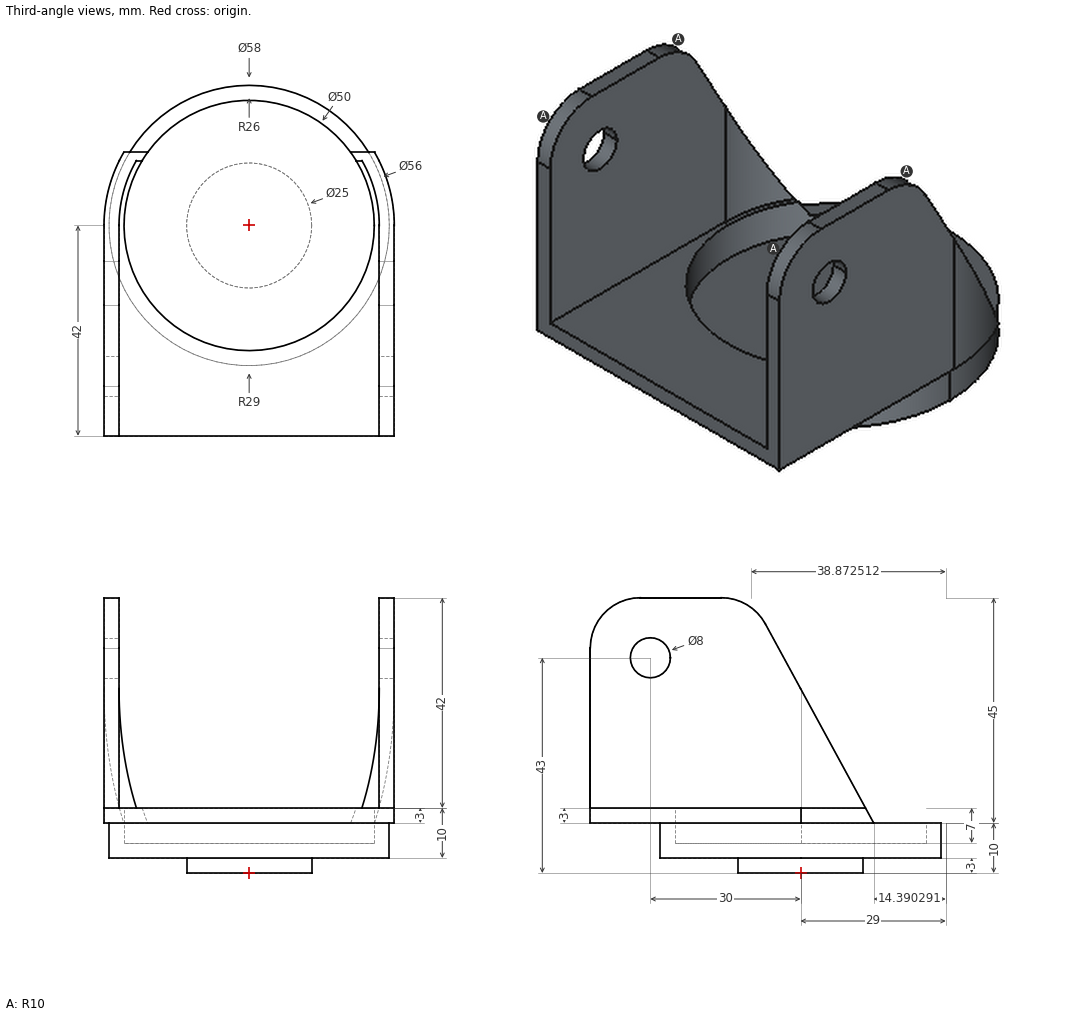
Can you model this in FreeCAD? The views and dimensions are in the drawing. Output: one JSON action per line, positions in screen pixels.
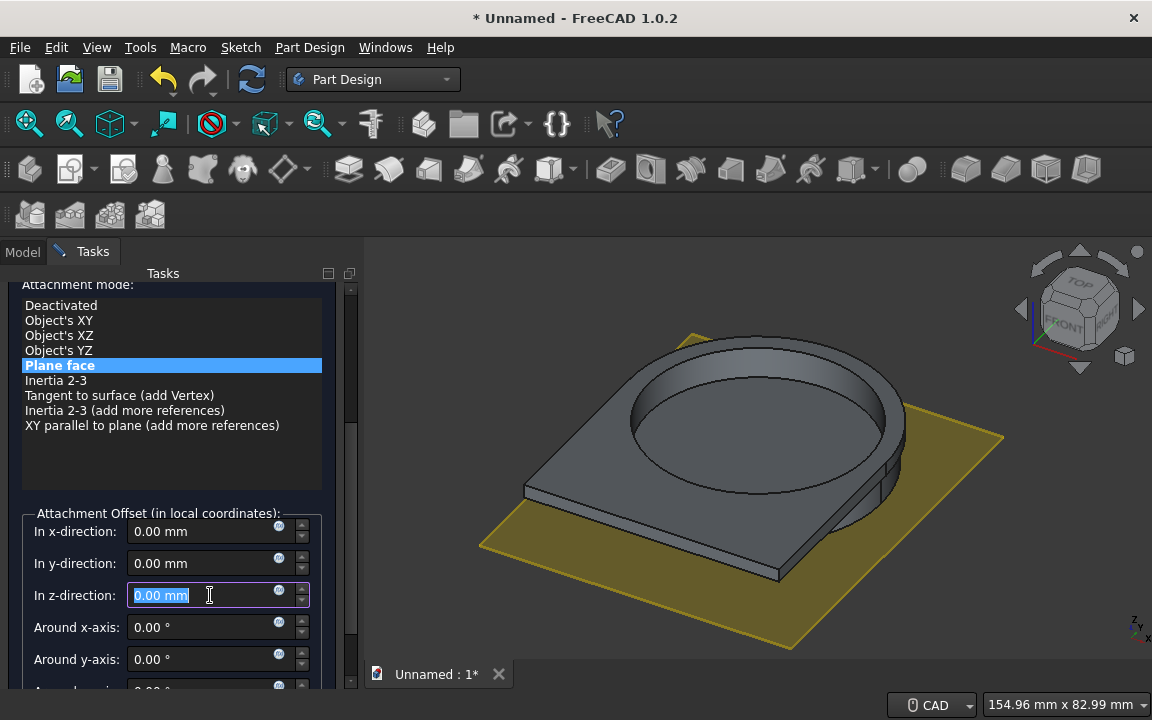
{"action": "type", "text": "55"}
{"action": "key", "text": "Tab"}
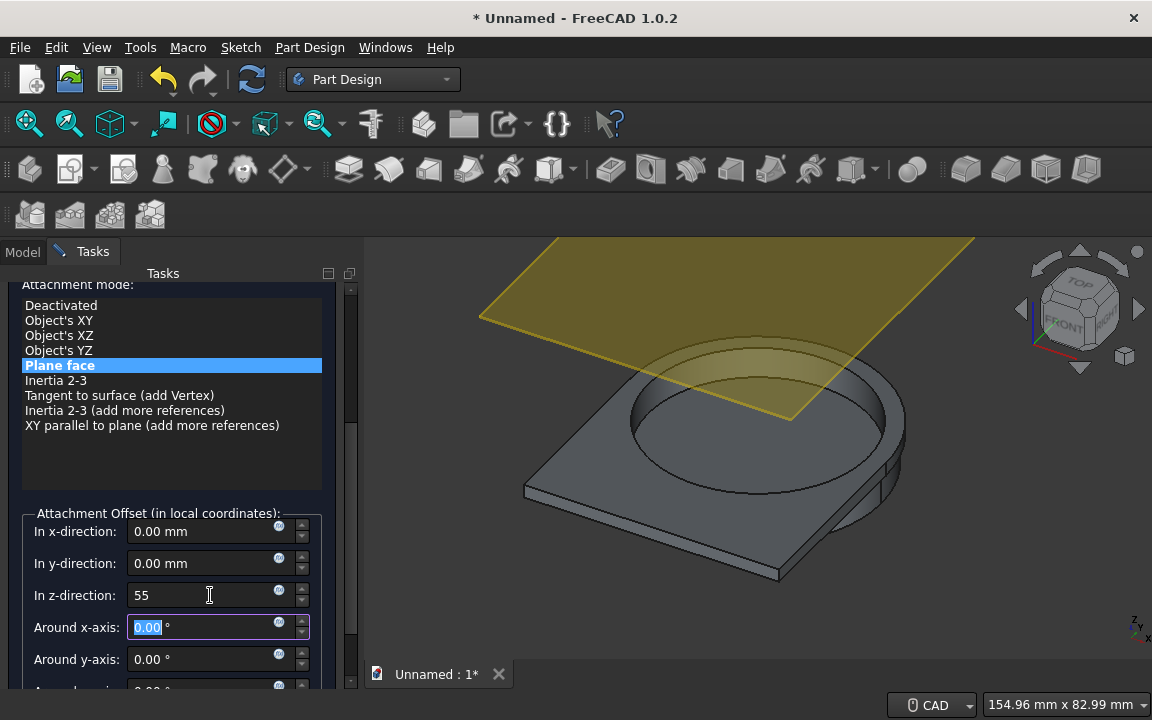
{"action": "scroll", "coordinate": [351, 486], "scroll_direction": "up", "scroll_amount": 5}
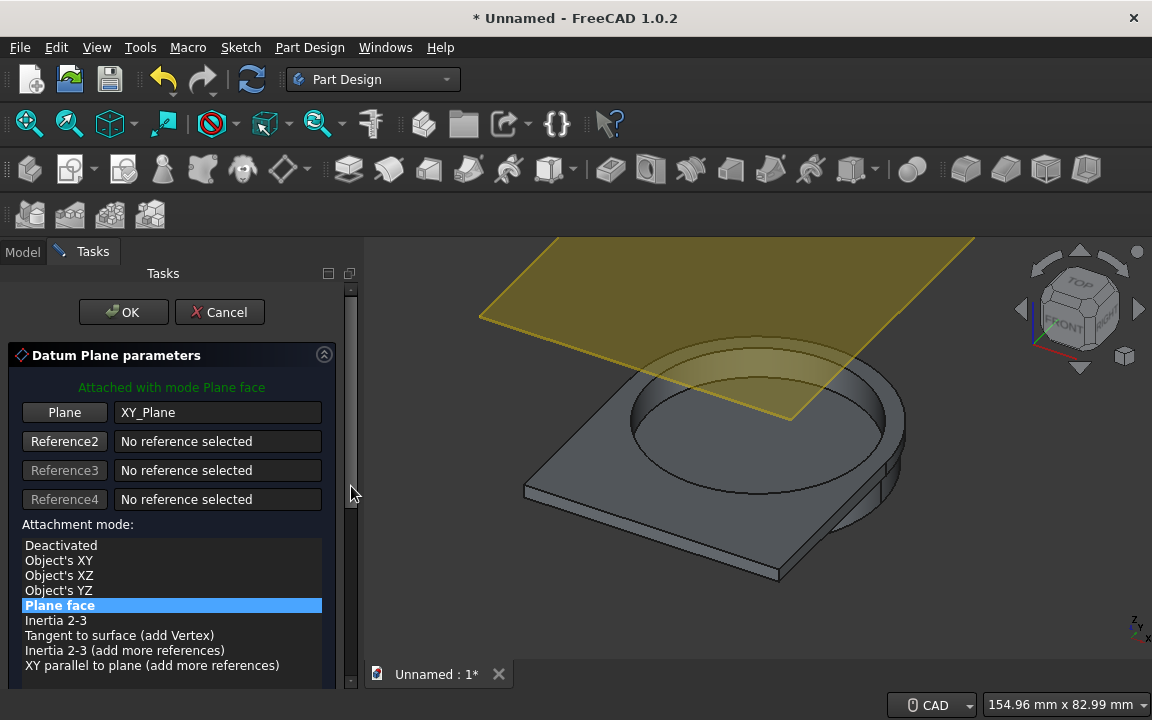
{"action": "left_click", "coordinate": [124, 312]}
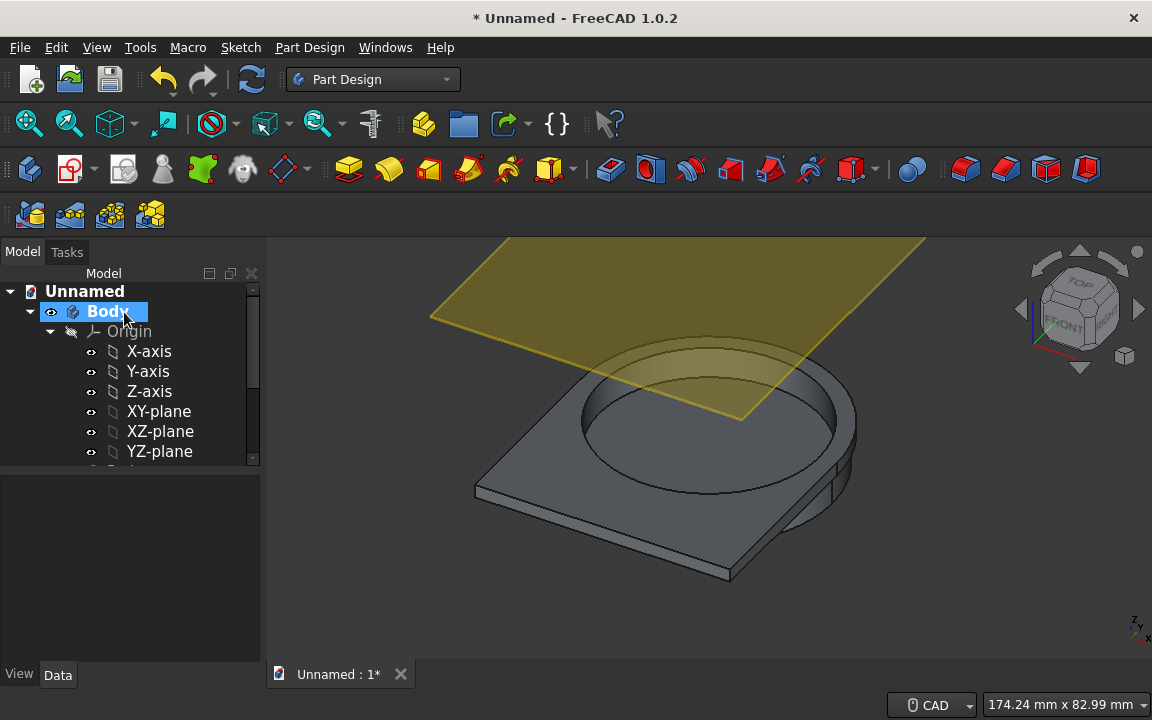
{"action": "scroll", "coordinate": [100, 367], "scroll_direction": "down", "scroll_amount": 3}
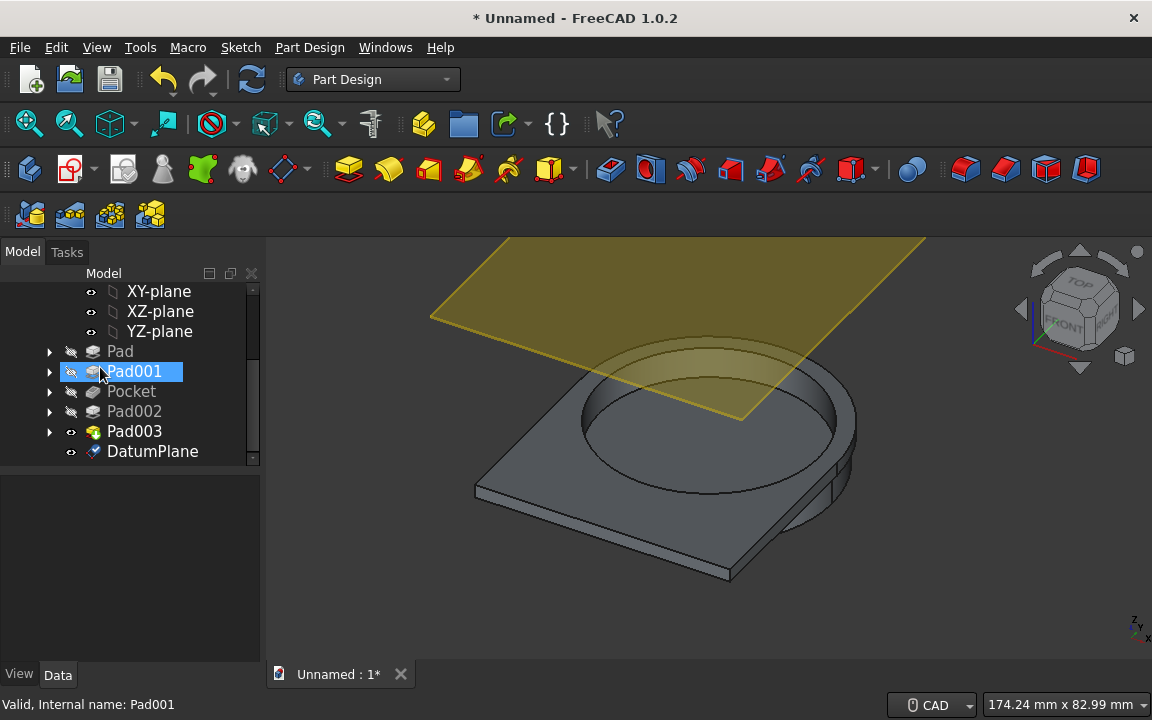
{"action": "left_click", "coordinate": [116, 452]}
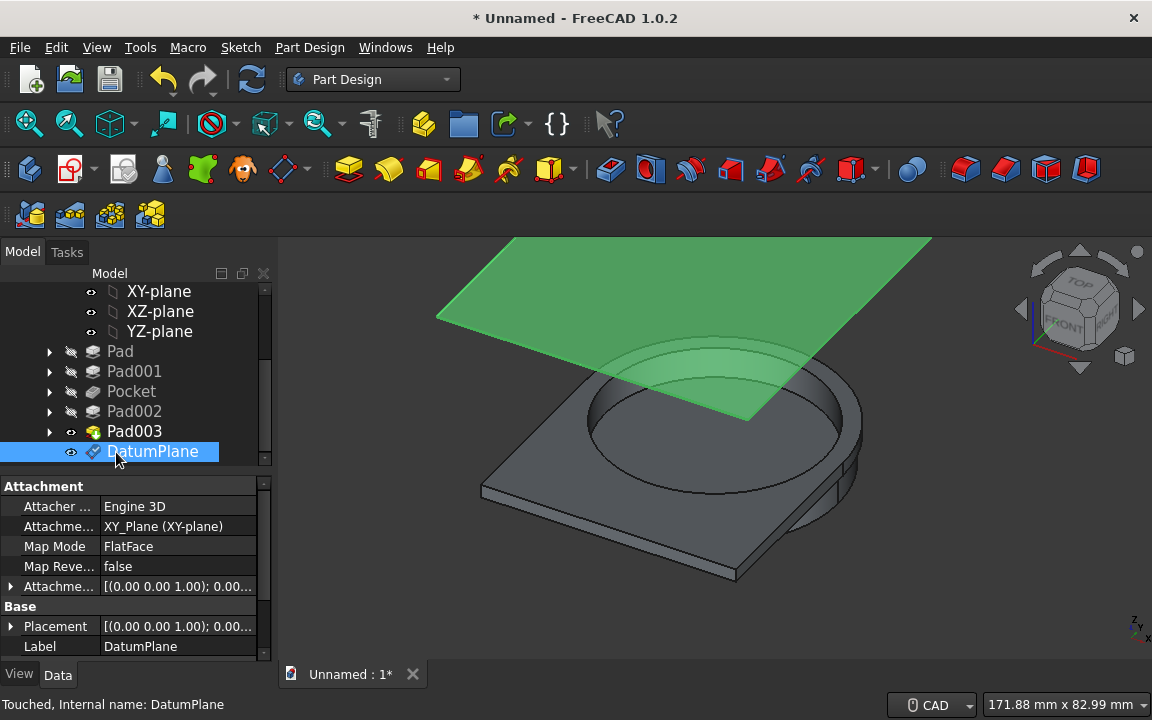
{"action": "left_click", "coordinate": [70, 170]}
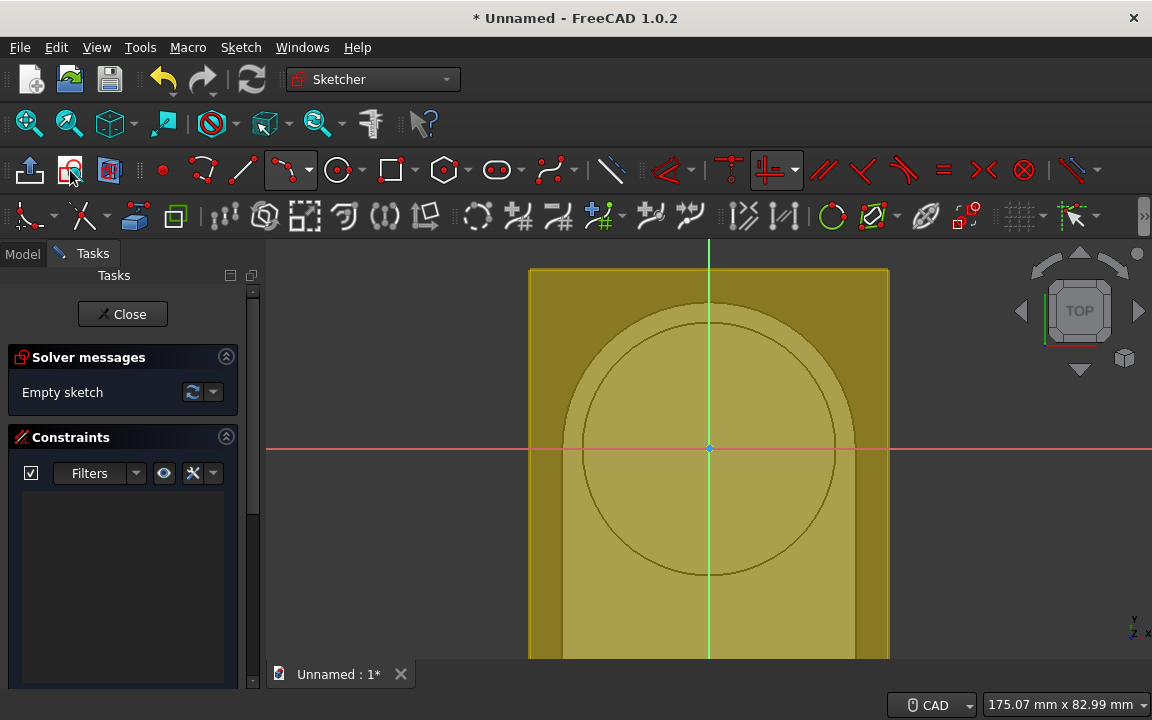
{"action": "scroll", "coordinate": [501, 382], "scroll_direction": "down", "scroll_amount": 2}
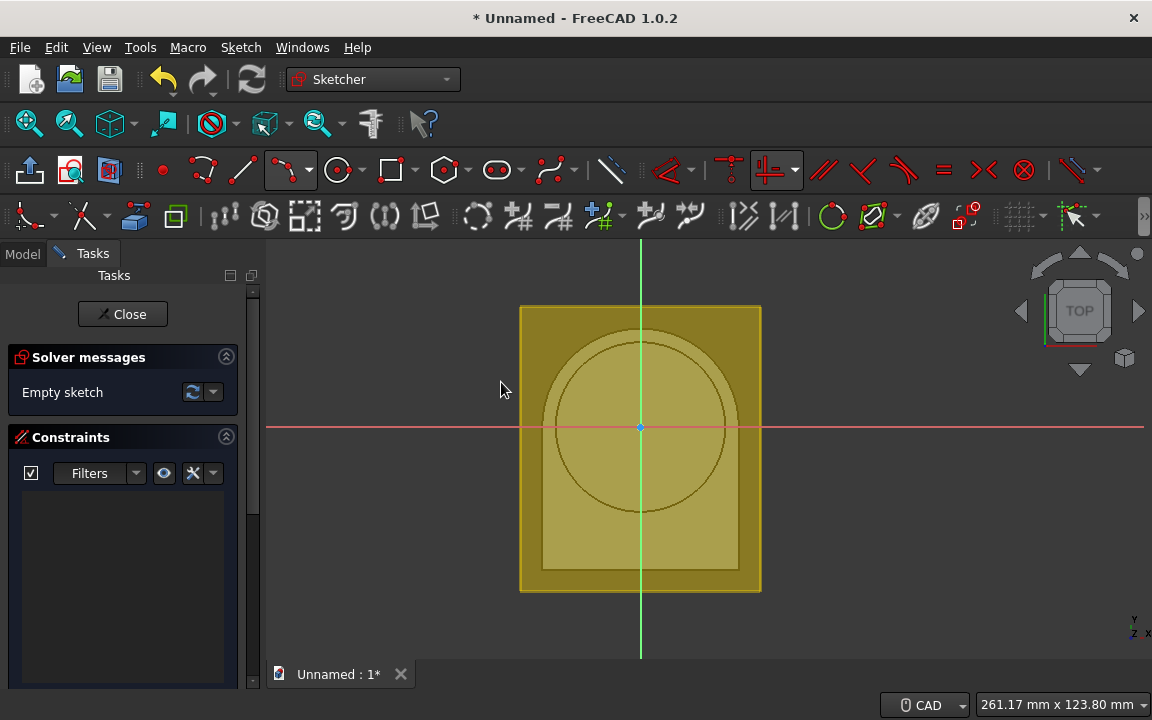
{"action": "left_click", "coordinate": [204, 170]}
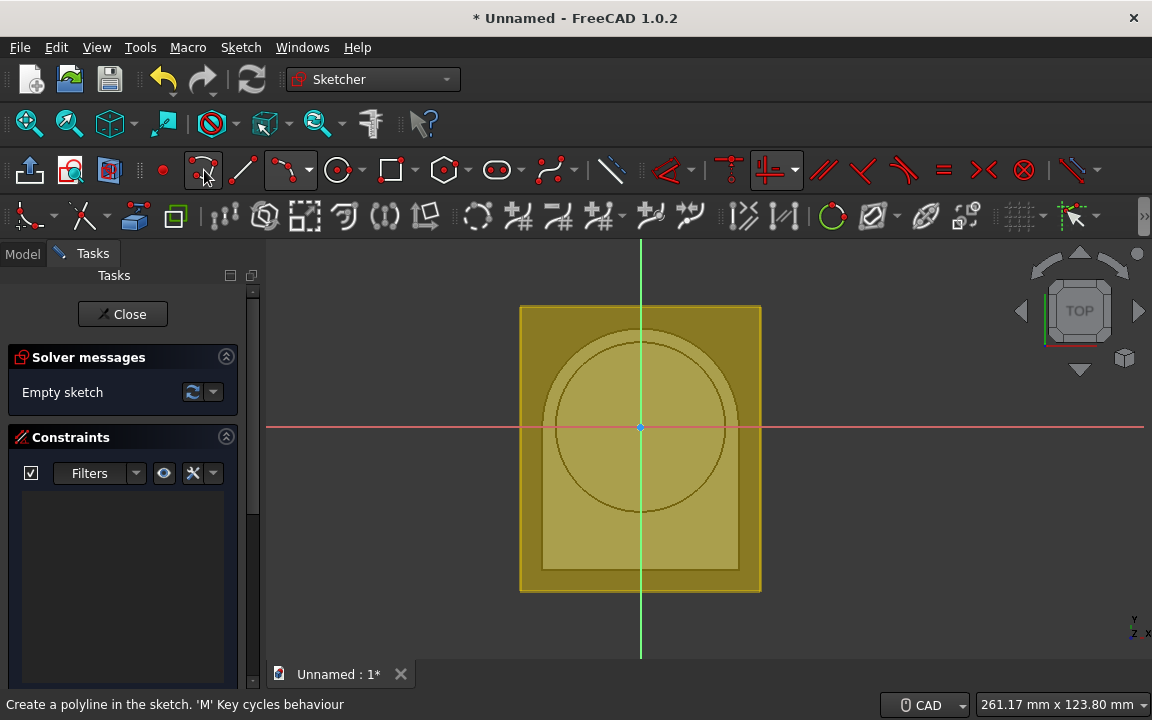
{"action": "left_click", "coordinate": [729, 427]}
{"action": "left_click", "coordinate": [729, 570]}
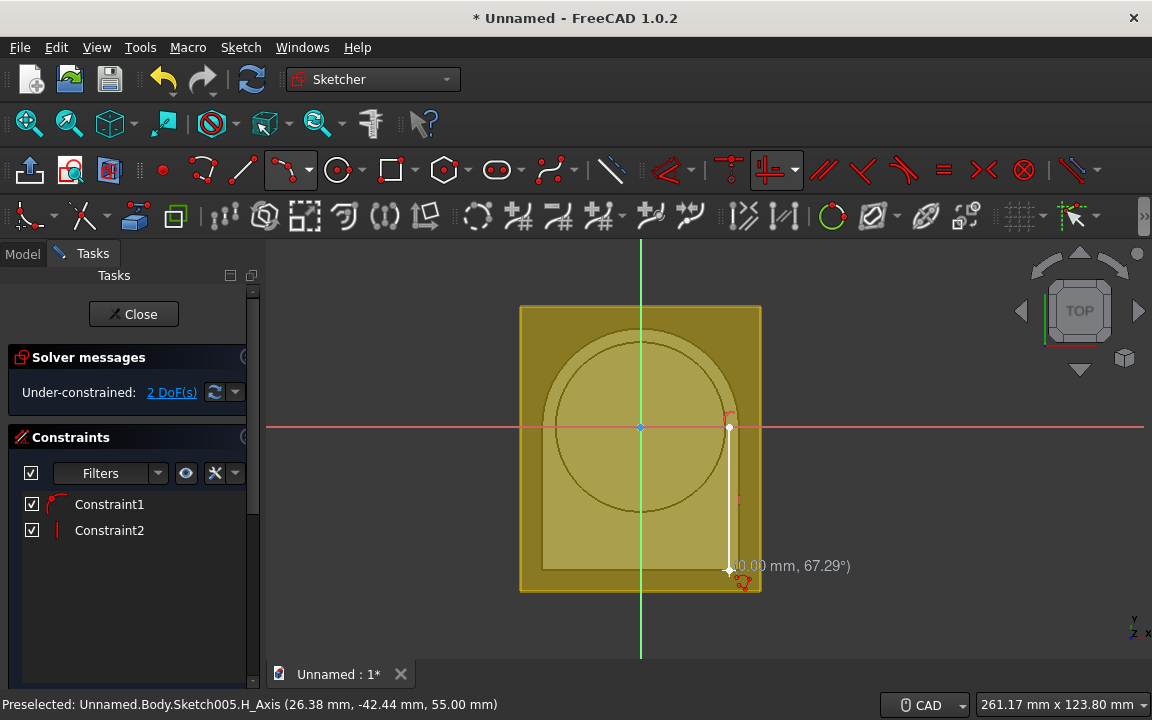
{"action": "scroll", "coordinate": [739, 570], "scroll_direction": "up", "scroll_amount": 3}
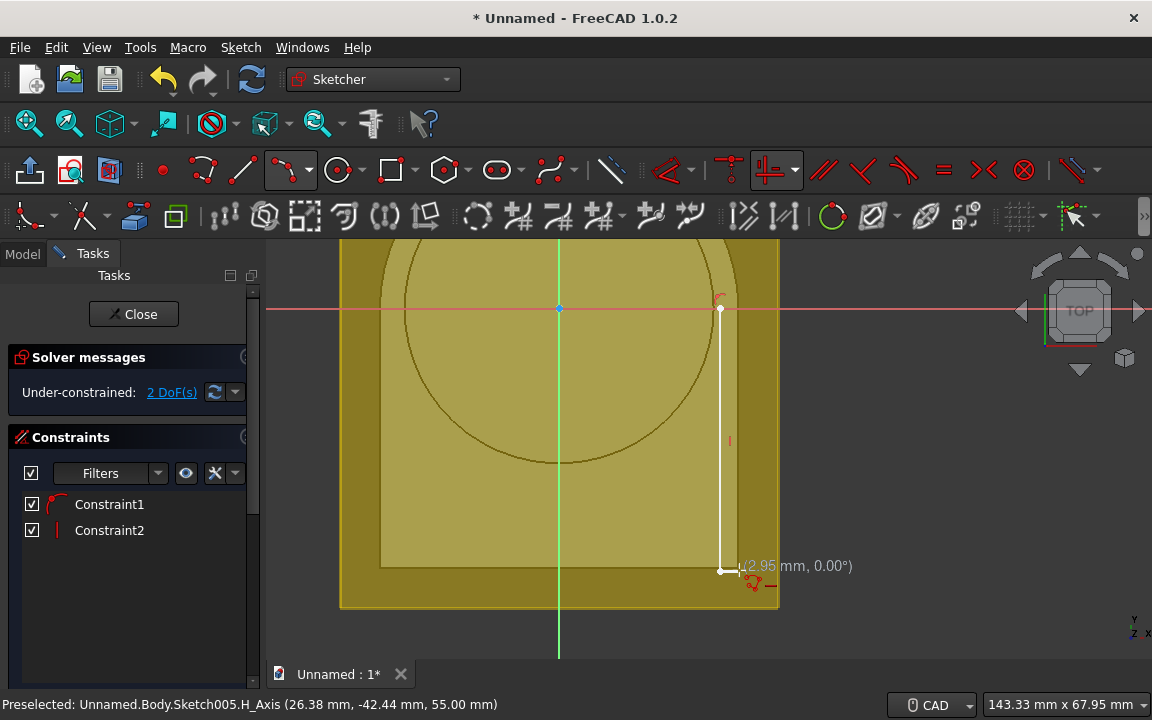
{"action": "left_click", "coordinate": [738, 569]}
{"action": "left_click", "coordinate": [738, 309]}
{"action": "right_click", "coordinate": [738, 309]}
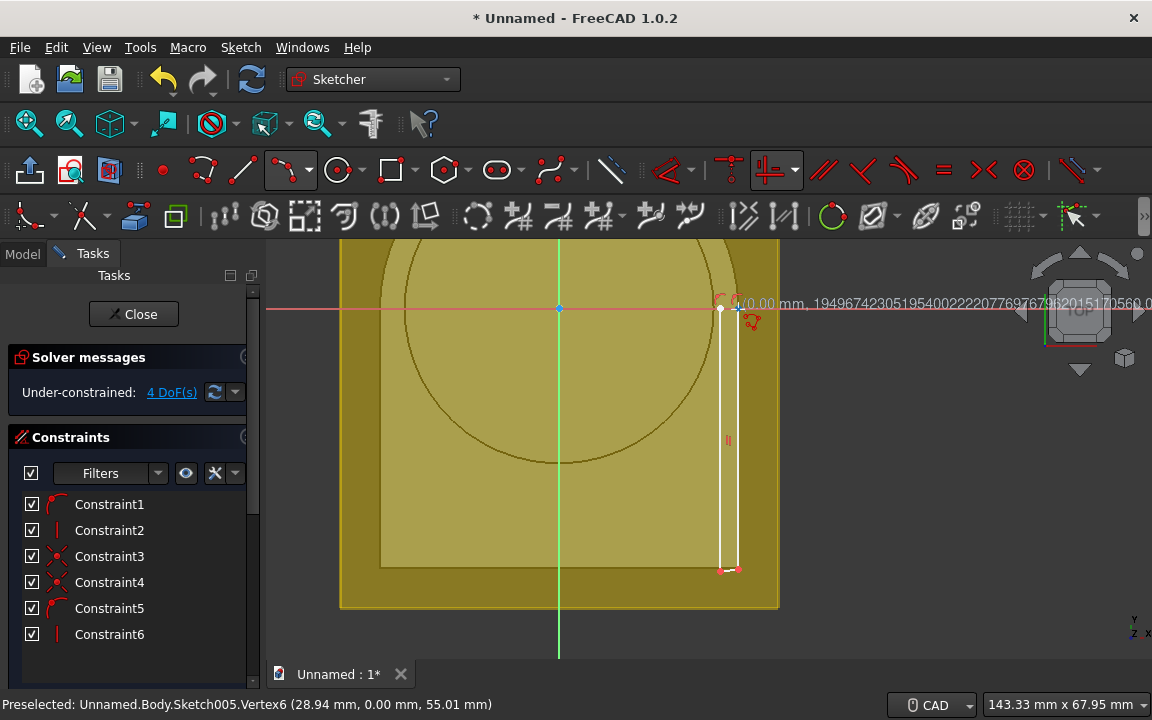
{"action": "left_click", "coordinate": [380, 309]}
{"action": "left_click", "coordinate": [380, 568]}
{"action": "left_click", "coordinate": [398, 568]}
{"action": "left_click", "coordinate": [398, 309]}
{"action": "right_click", "coordinate": [398, 309]}